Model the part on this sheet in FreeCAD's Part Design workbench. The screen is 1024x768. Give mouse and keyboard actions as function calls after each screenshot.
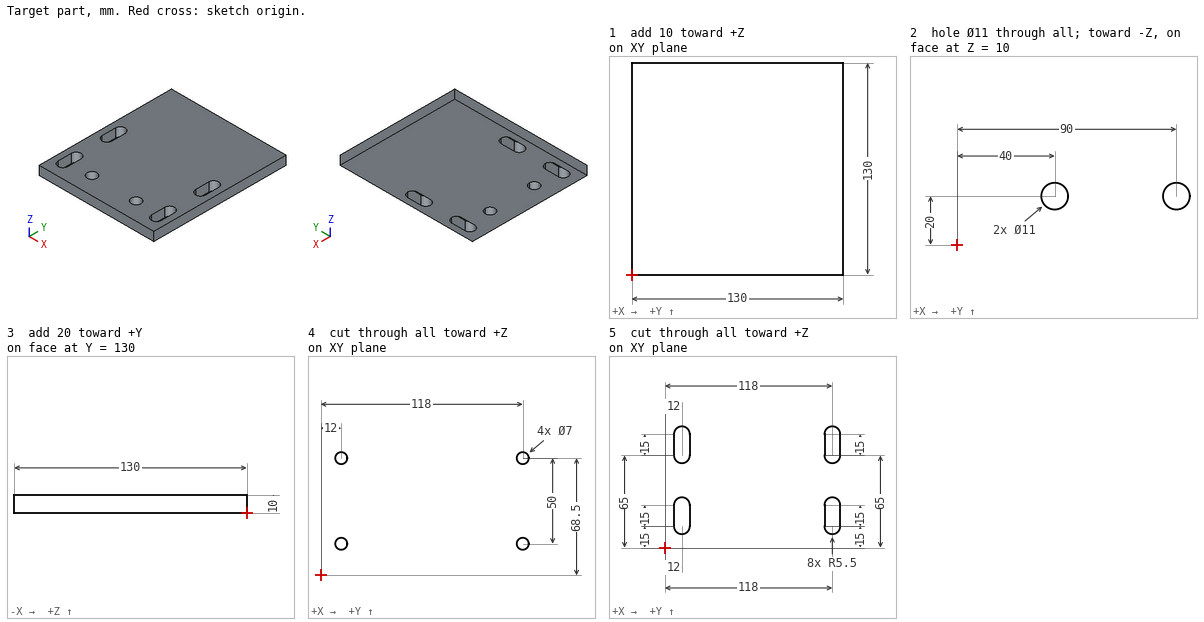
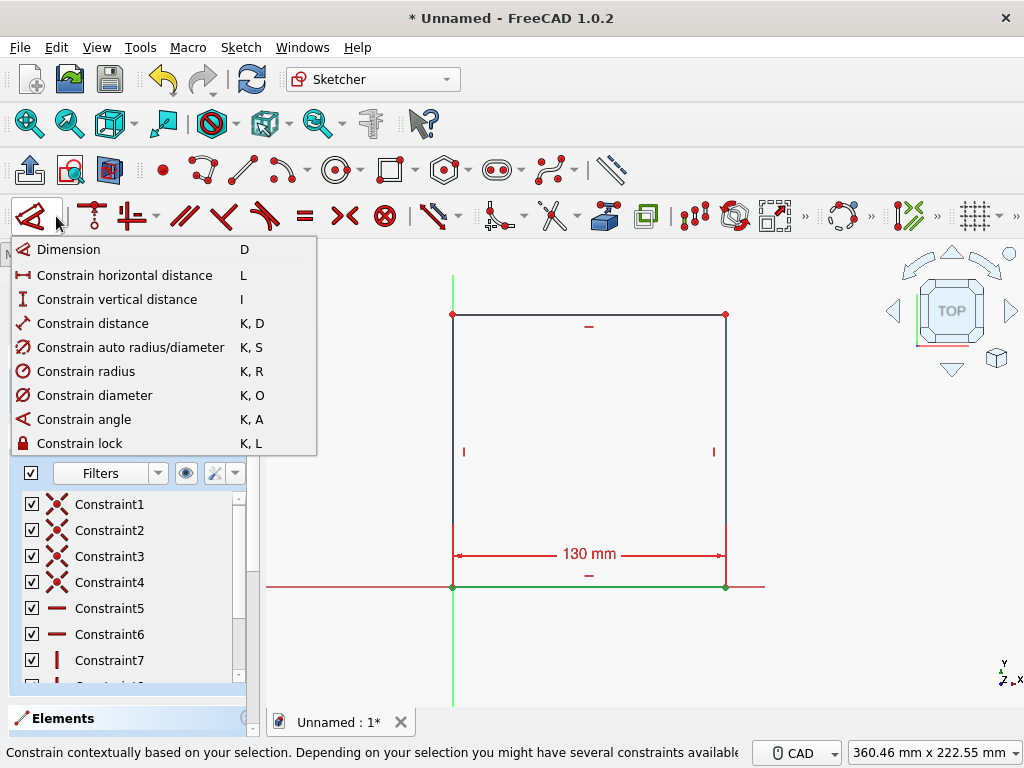
click(164, 299)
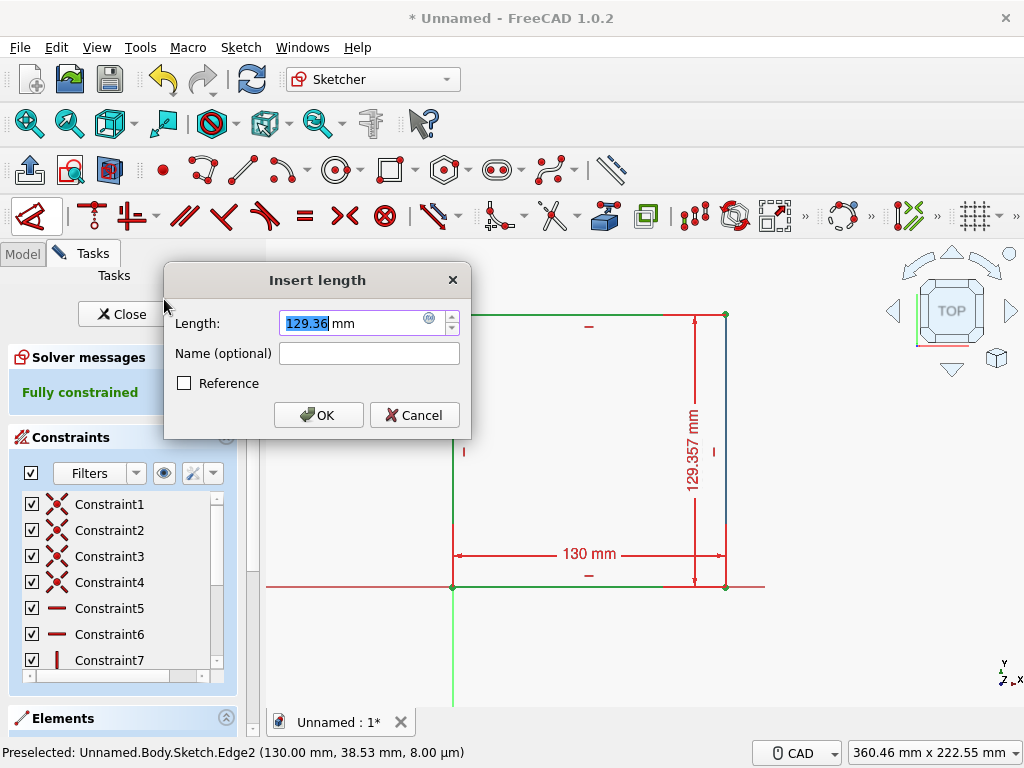
text(130)
key(Return)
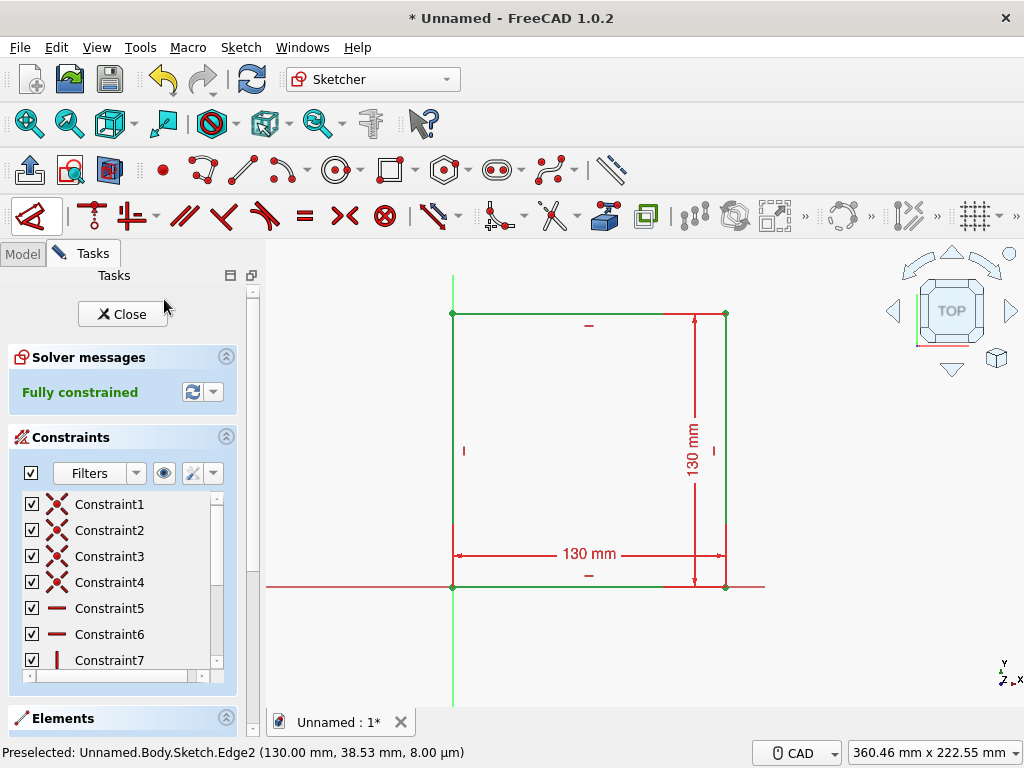
click(123, 314)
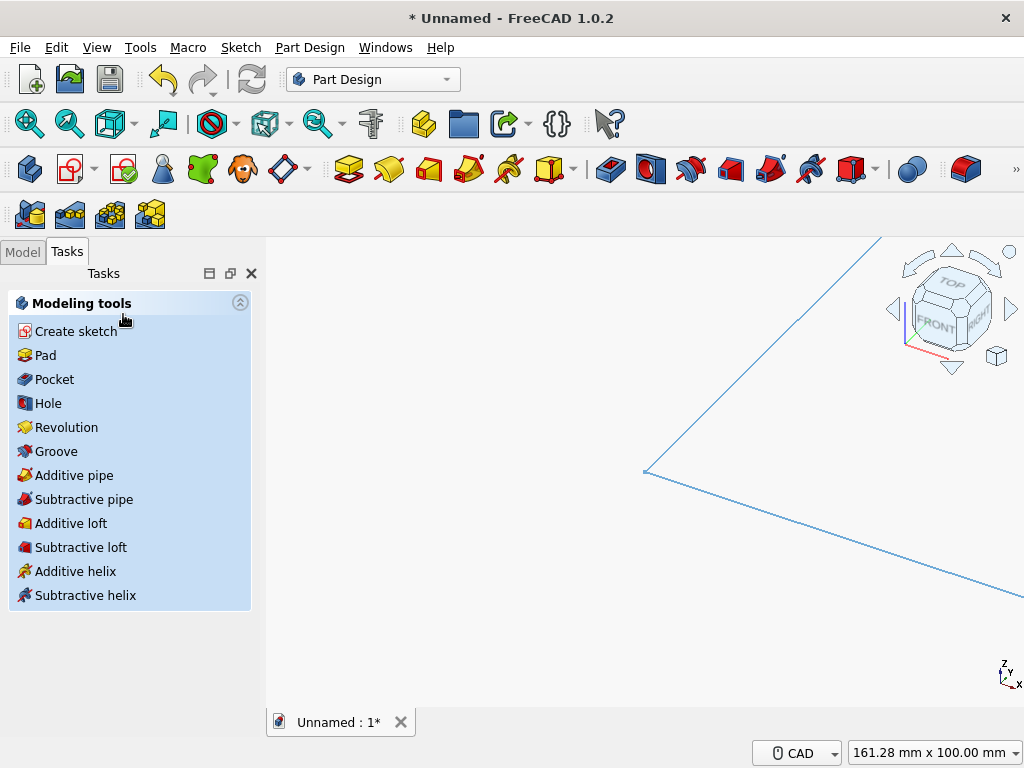
click(350, 170)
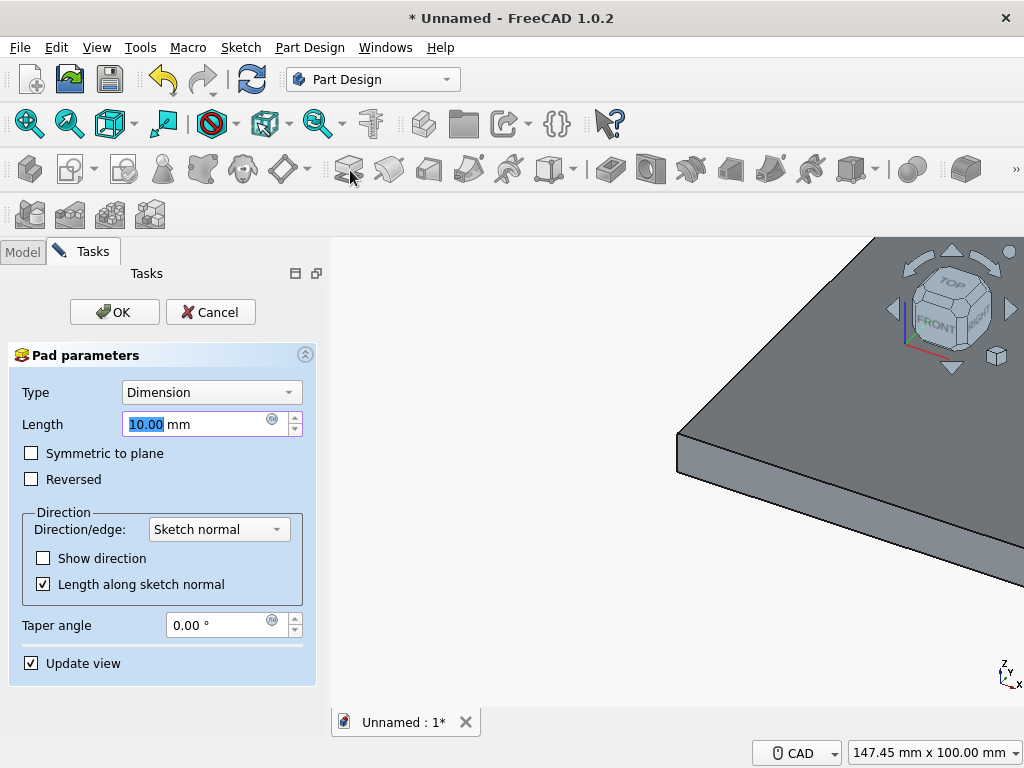
text(10)
key(Tab)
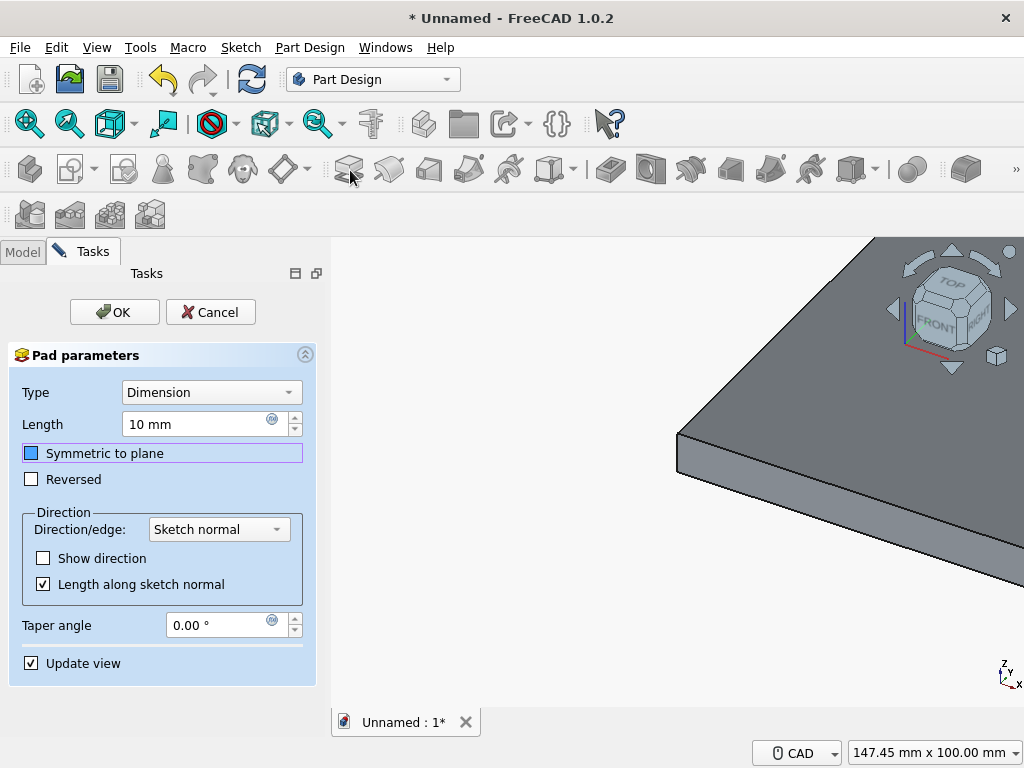
click(115, 312)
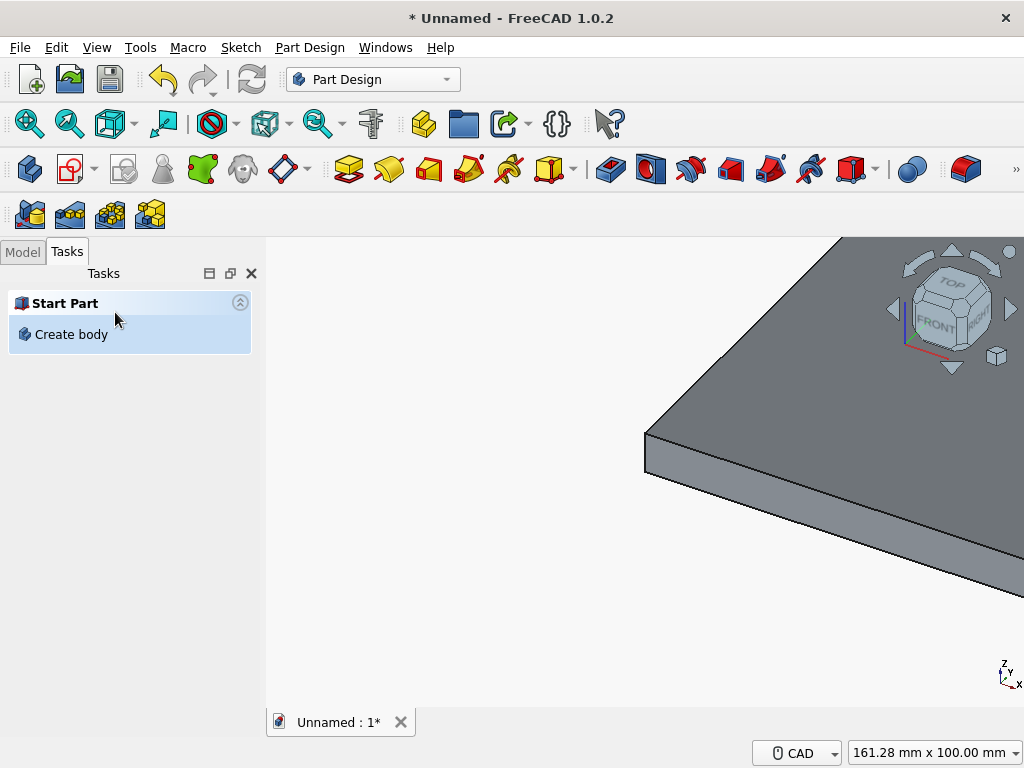
click(30, 124)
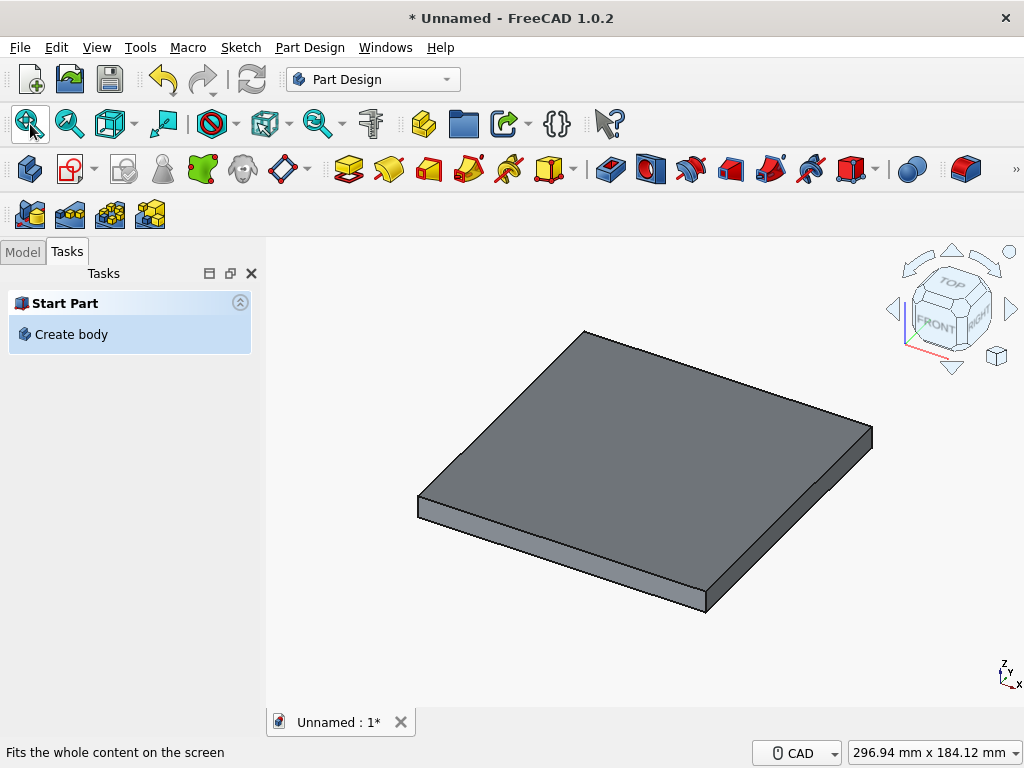
click(645, 461)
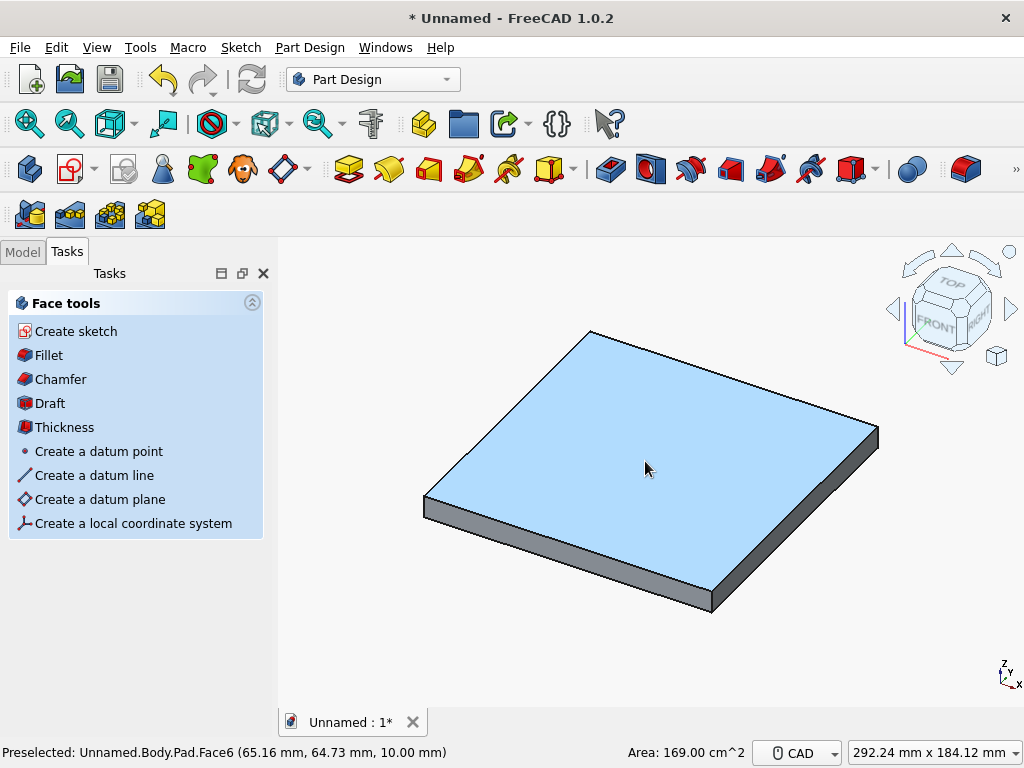
click(70, 170)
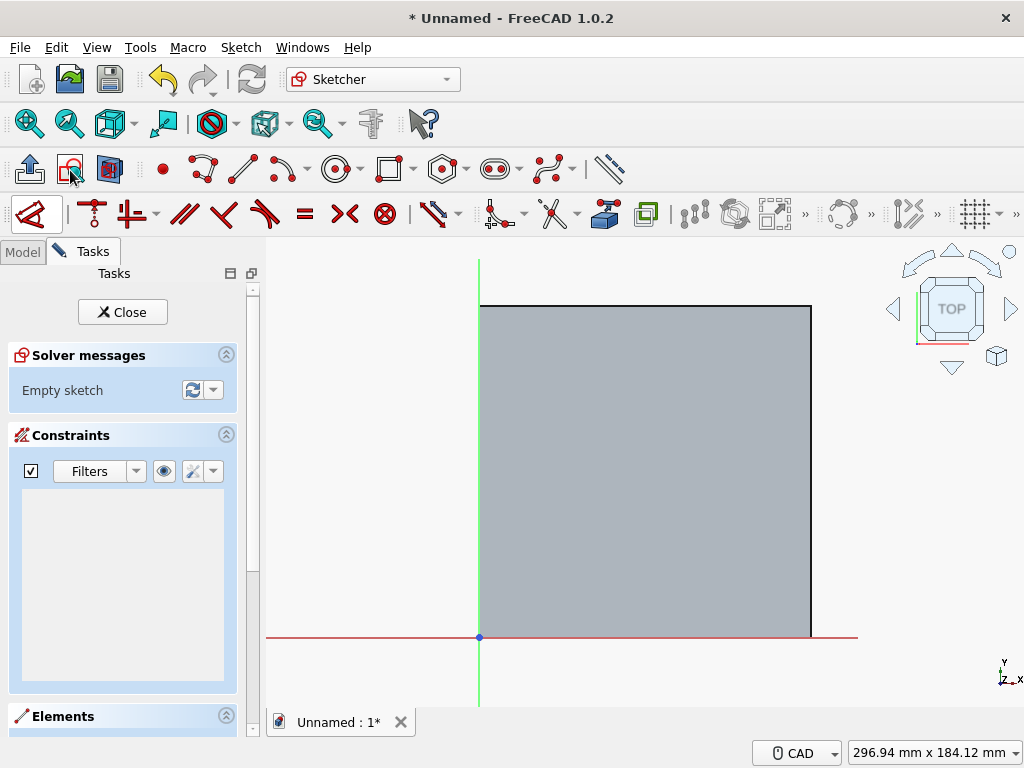
scroll(651, 679, up, 2)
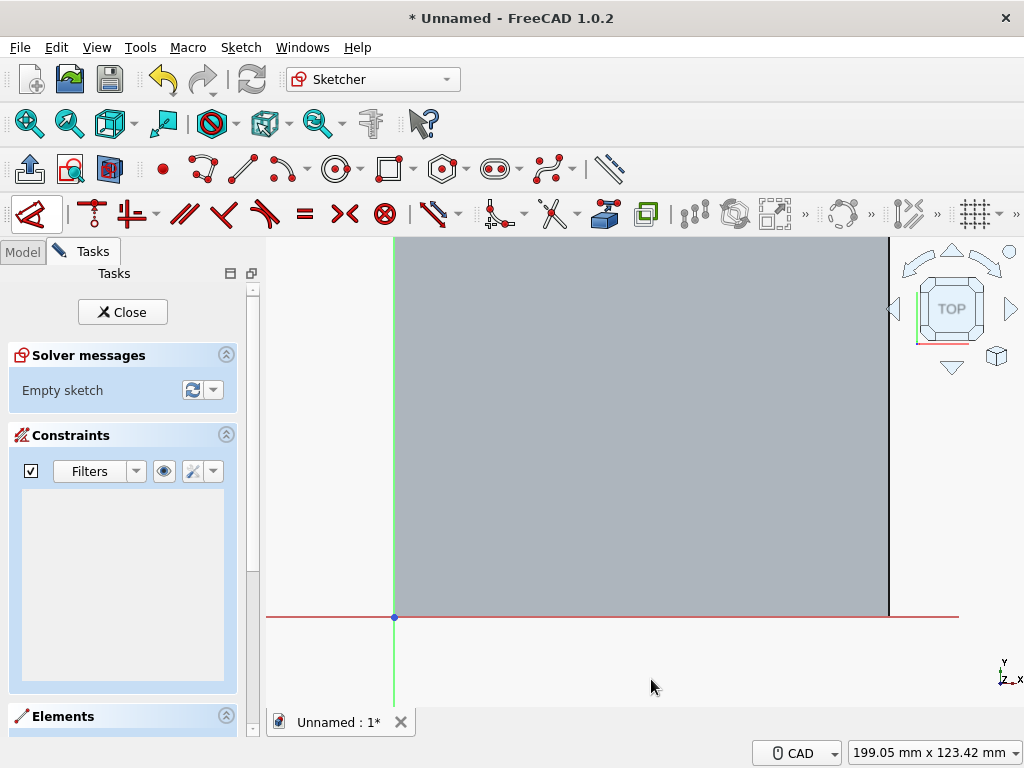
click(336, 170)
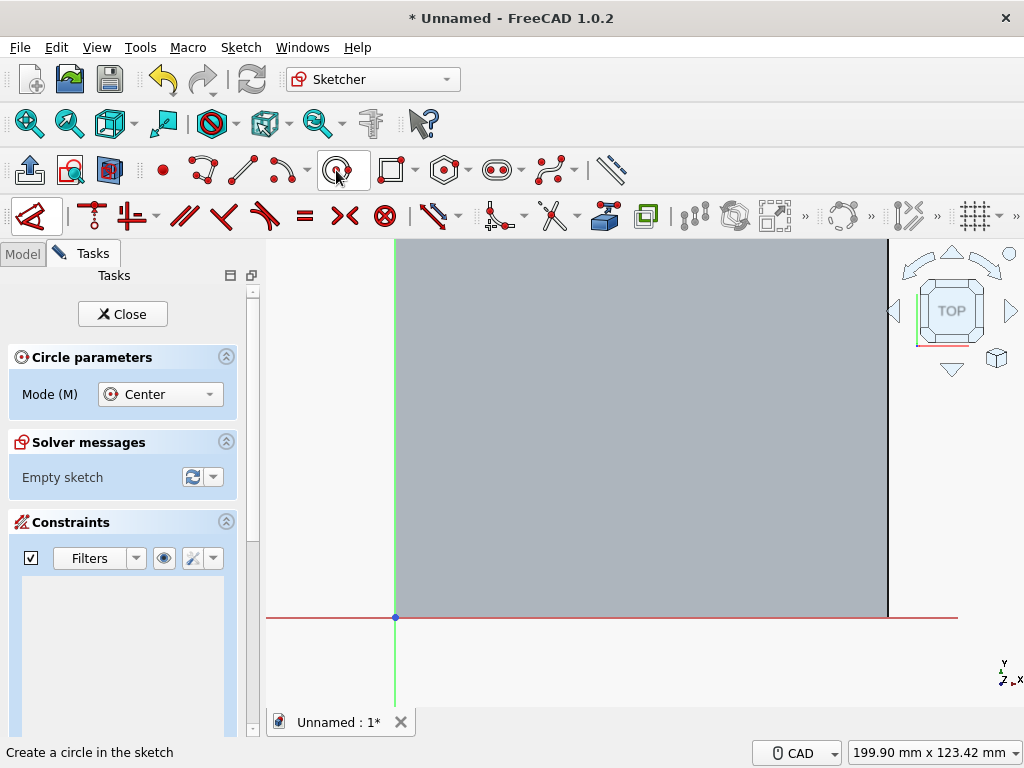
click(547, 542)
click(562, 527)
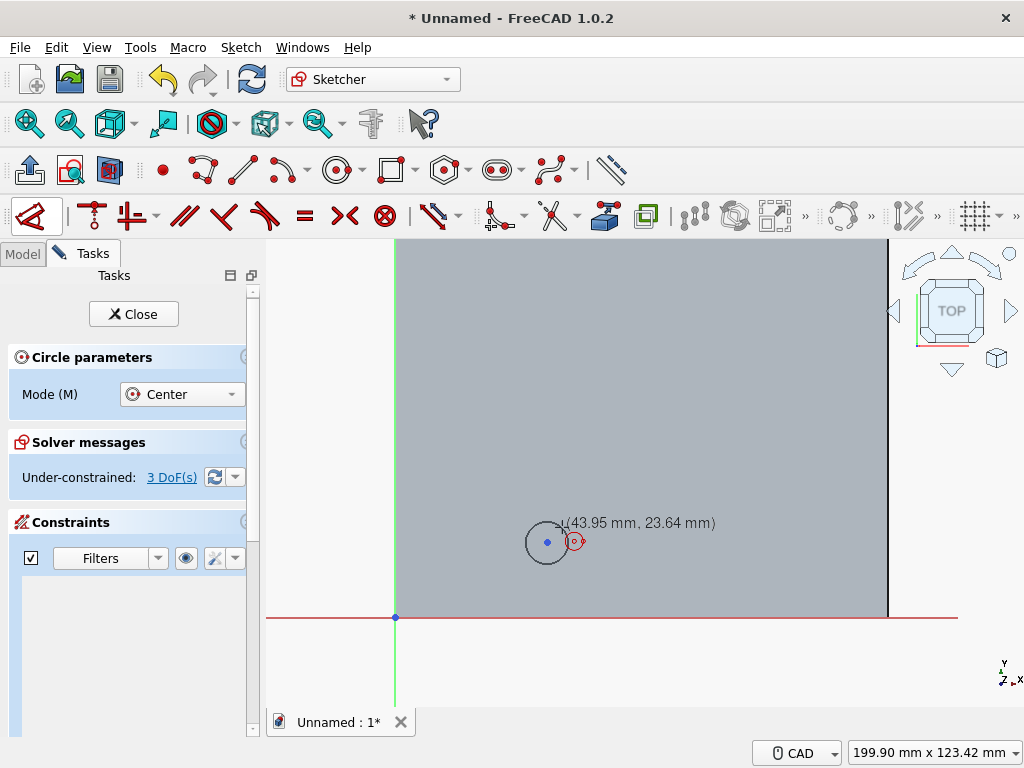
click(737, 542)
click(751, 527)
key(Escape)